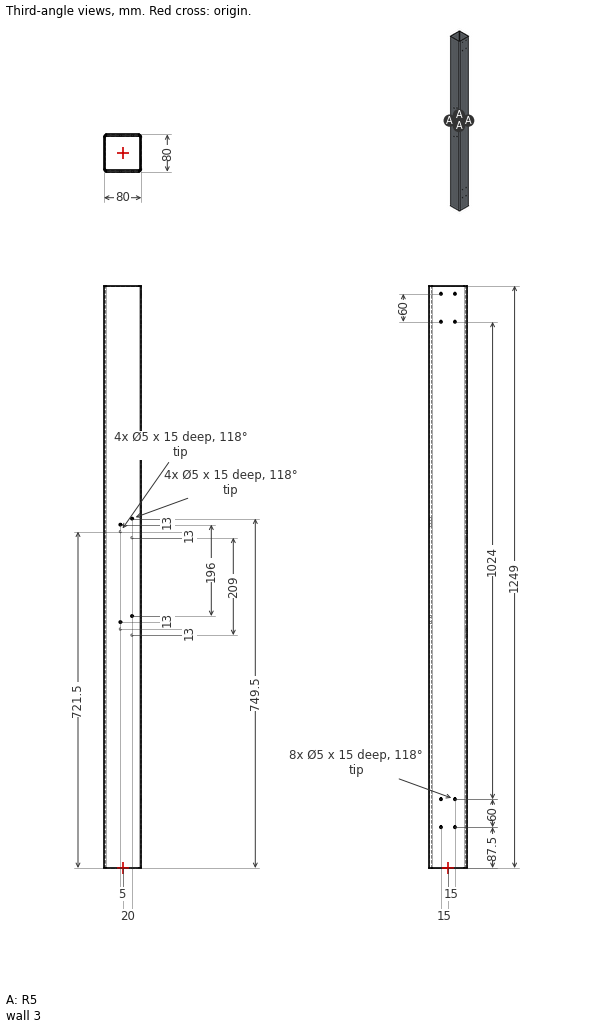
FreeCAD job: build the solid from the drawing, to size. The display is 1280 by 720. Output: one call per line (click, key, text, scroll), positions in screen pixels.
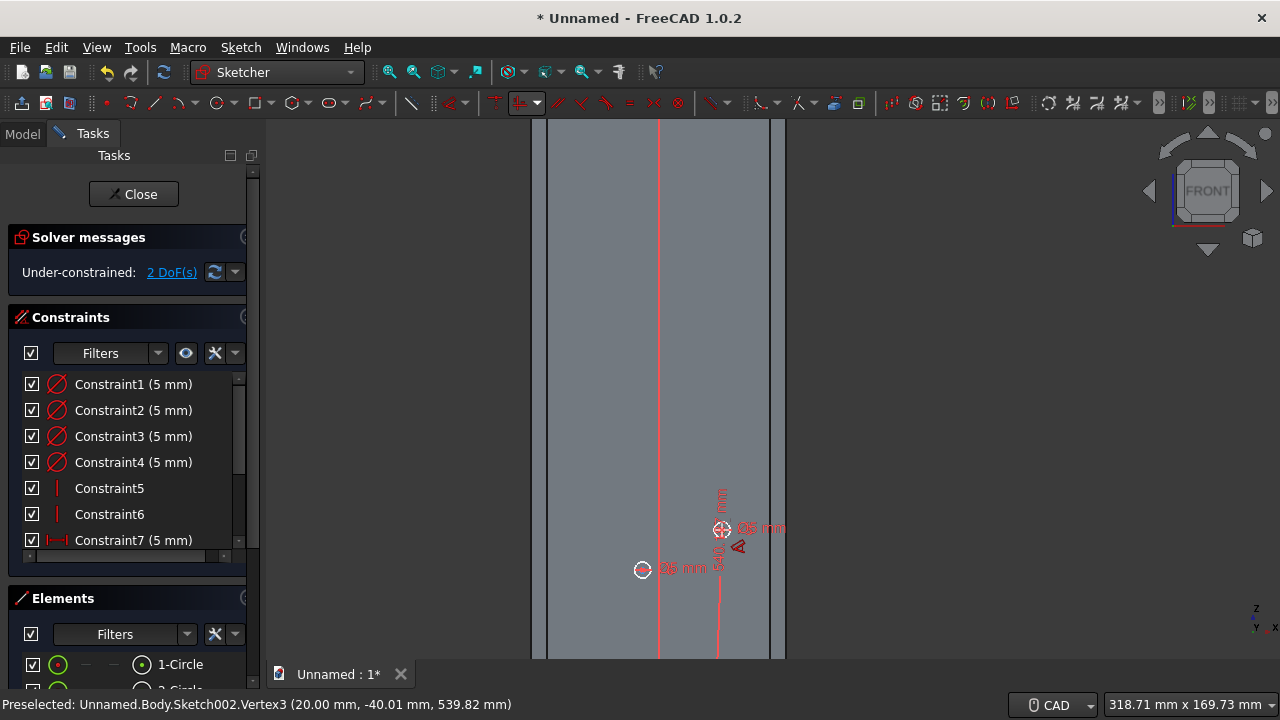
click(643, 570)
click(756, 550)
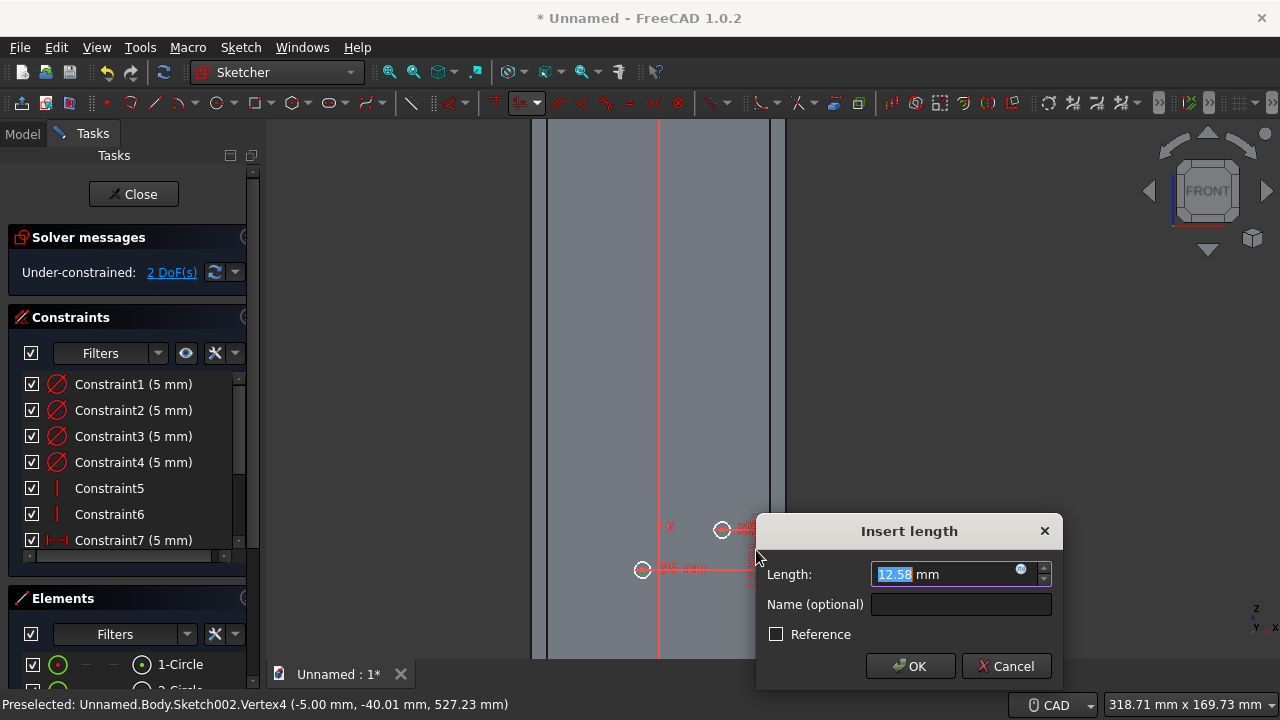
text(13)
key(Return)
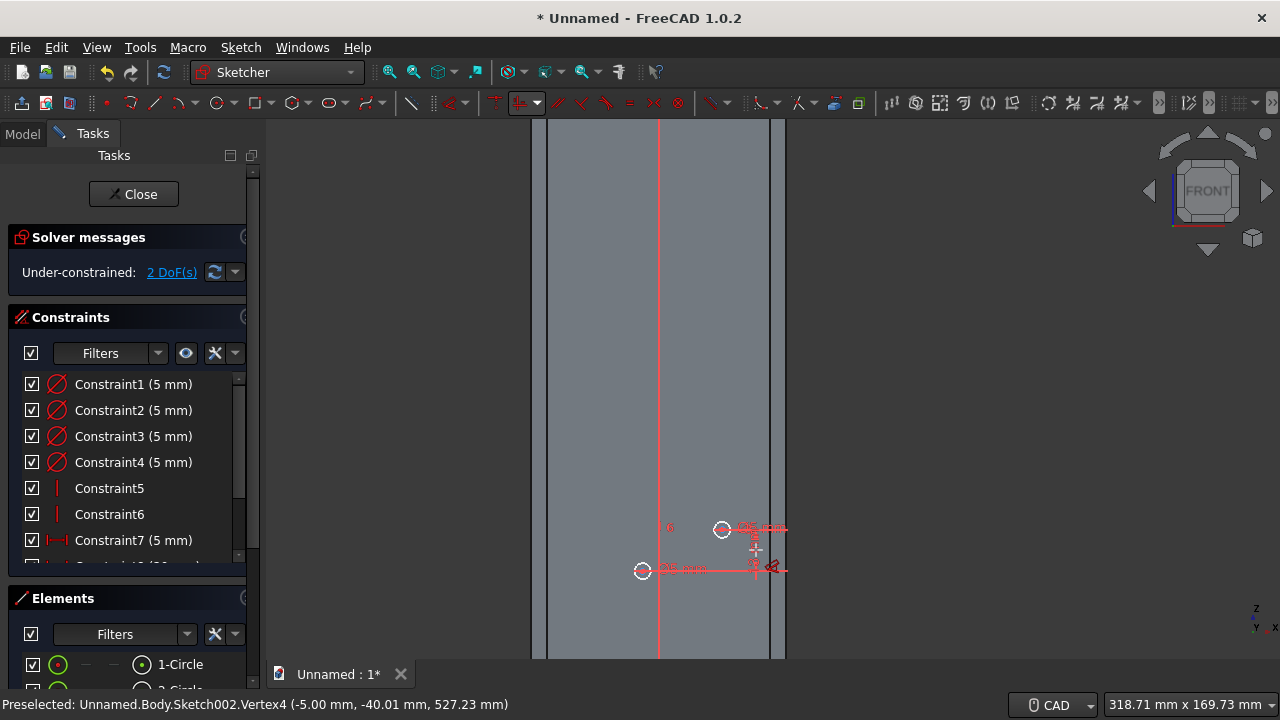
scroll(723, 530, down, 4)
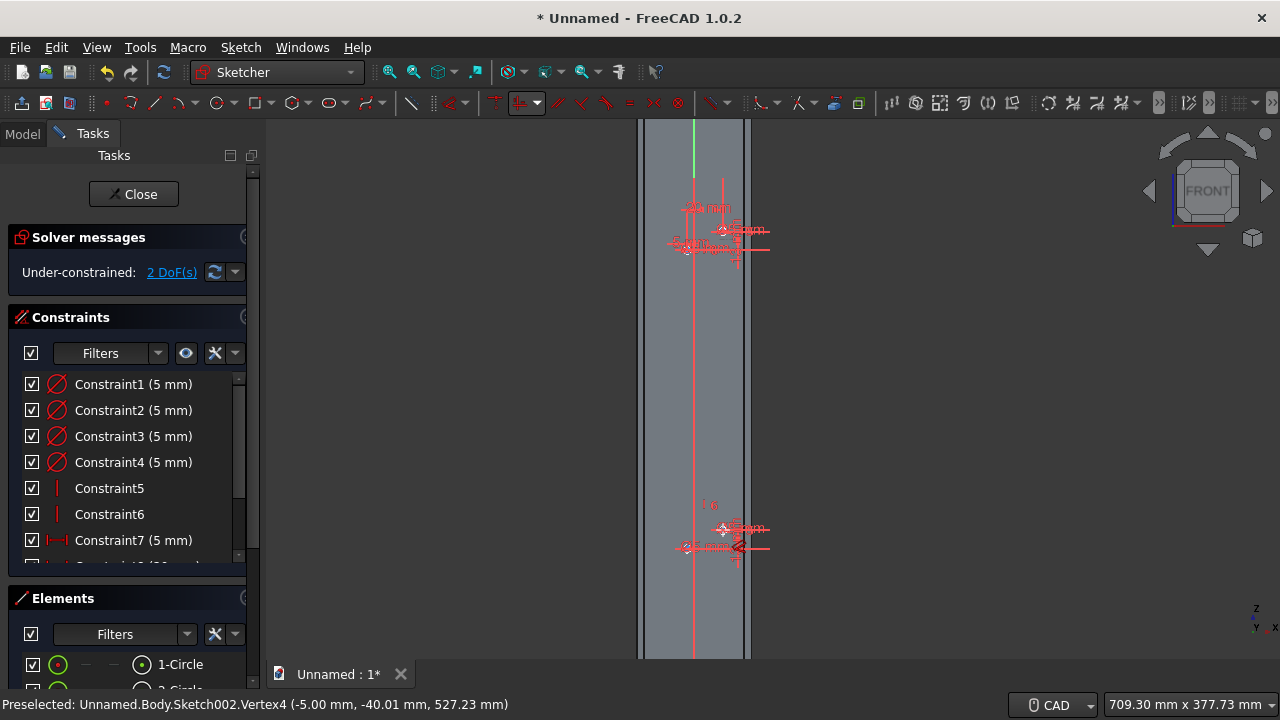
click(687, 250)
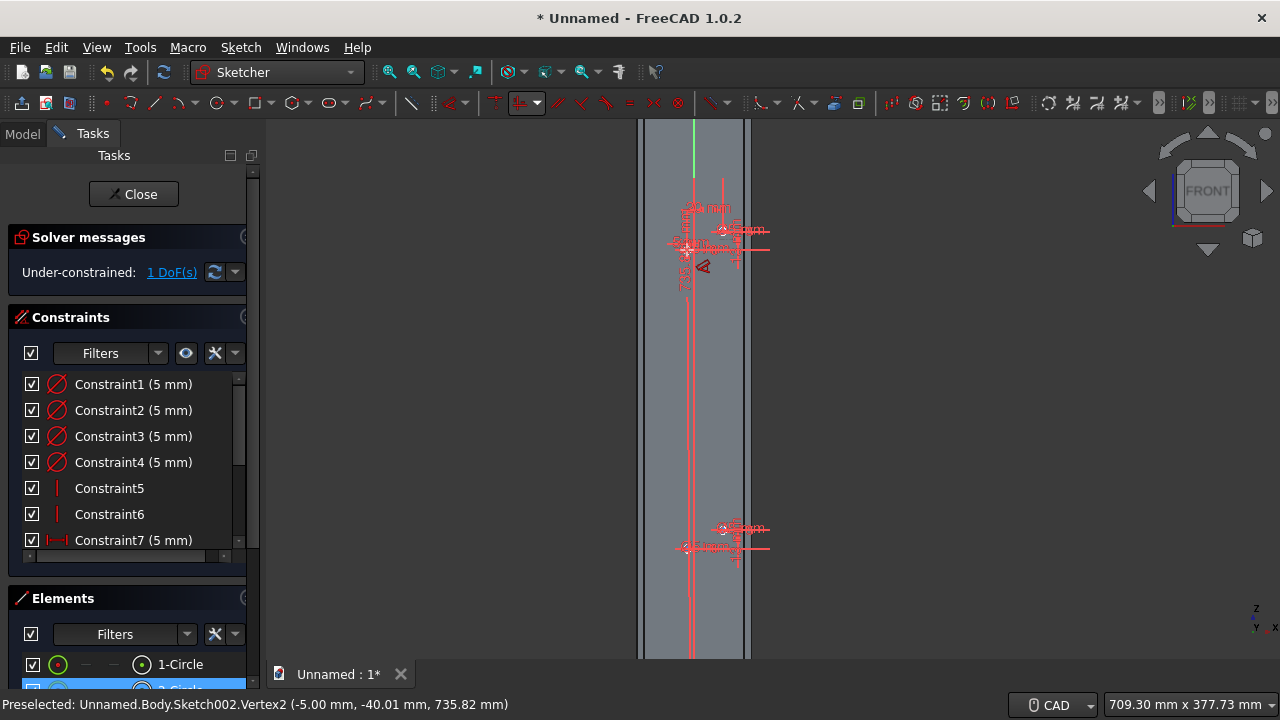
click(723, 530)
click(757, 390)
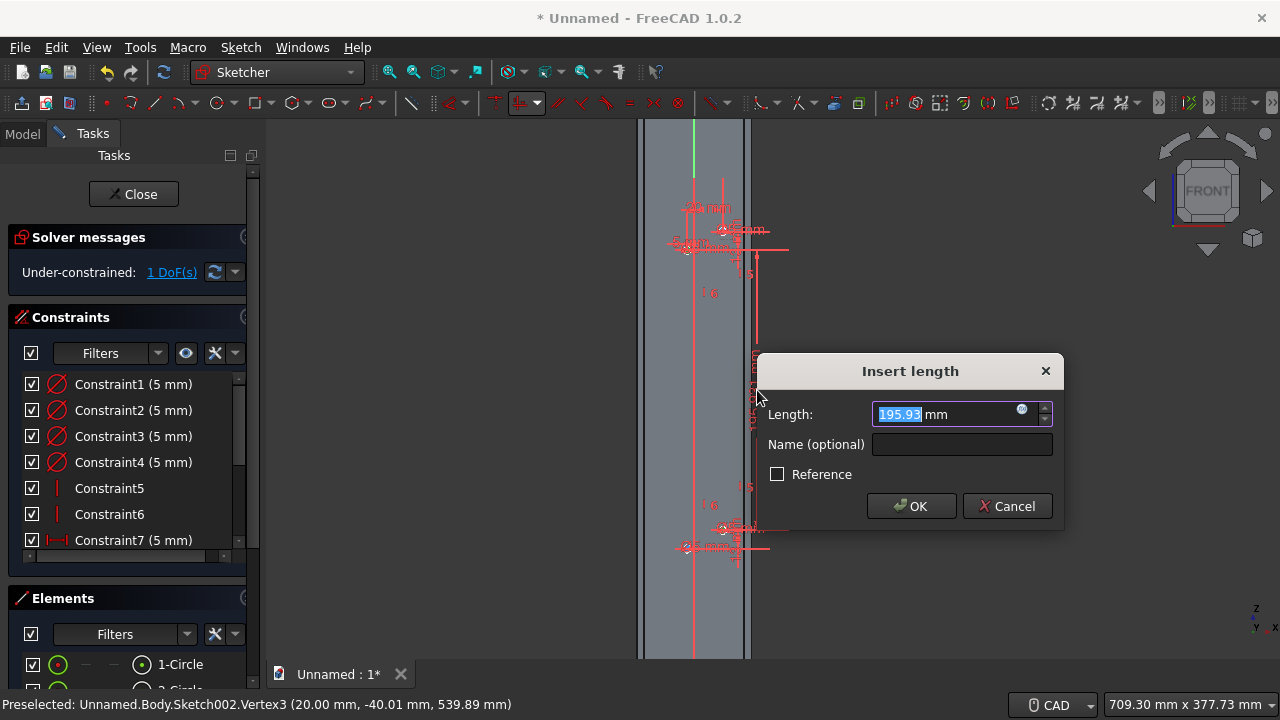
text(196)
key(Return)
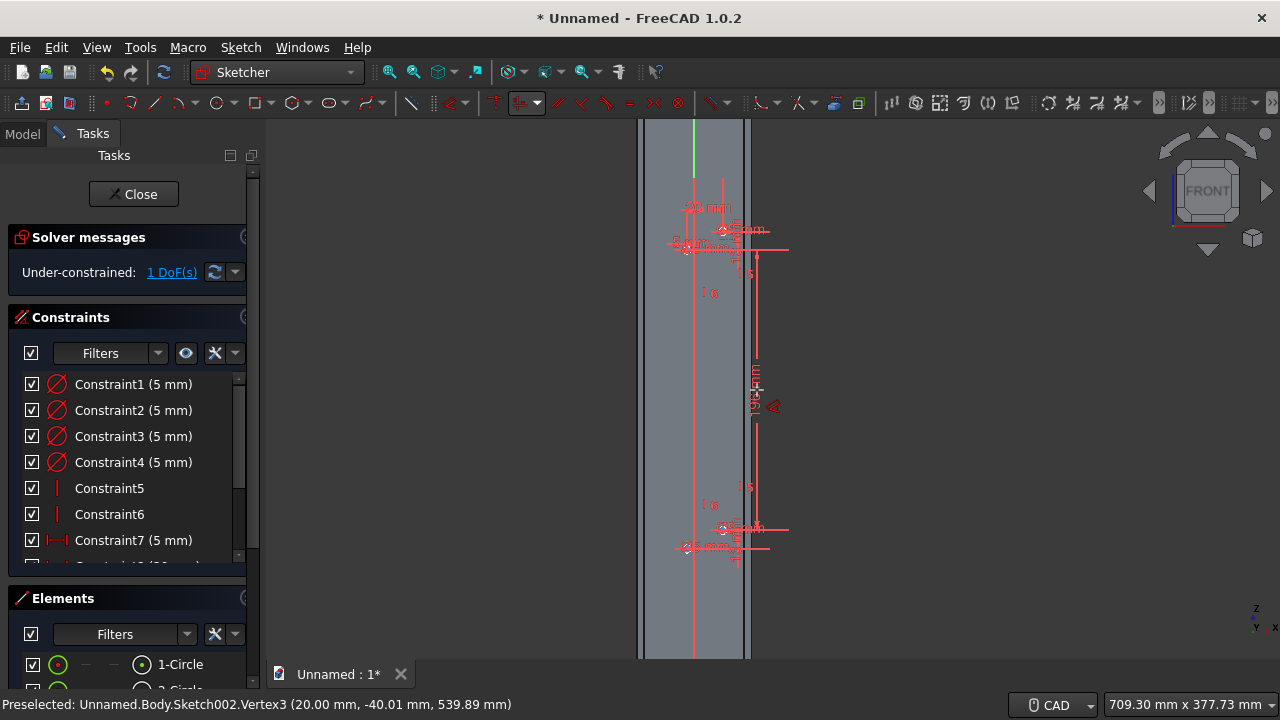
click(723, 232)
click(757, 431)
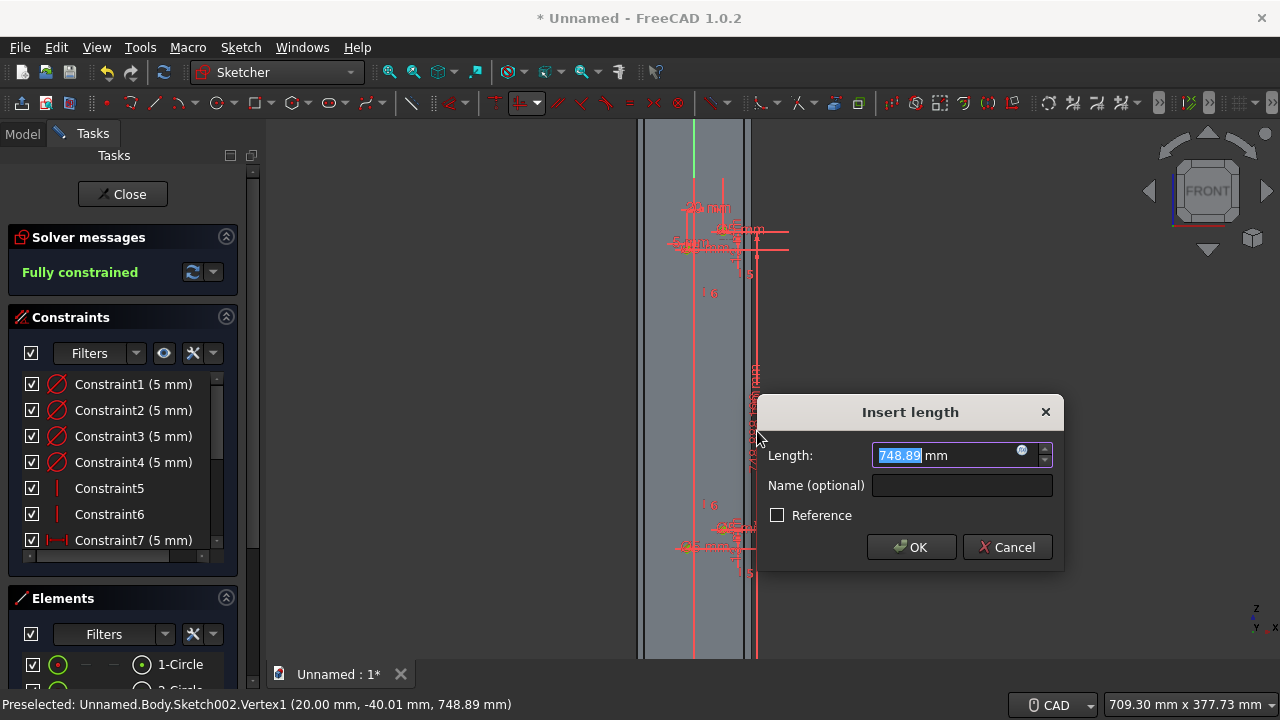
text(749.5)
key(Return)
key(Escape)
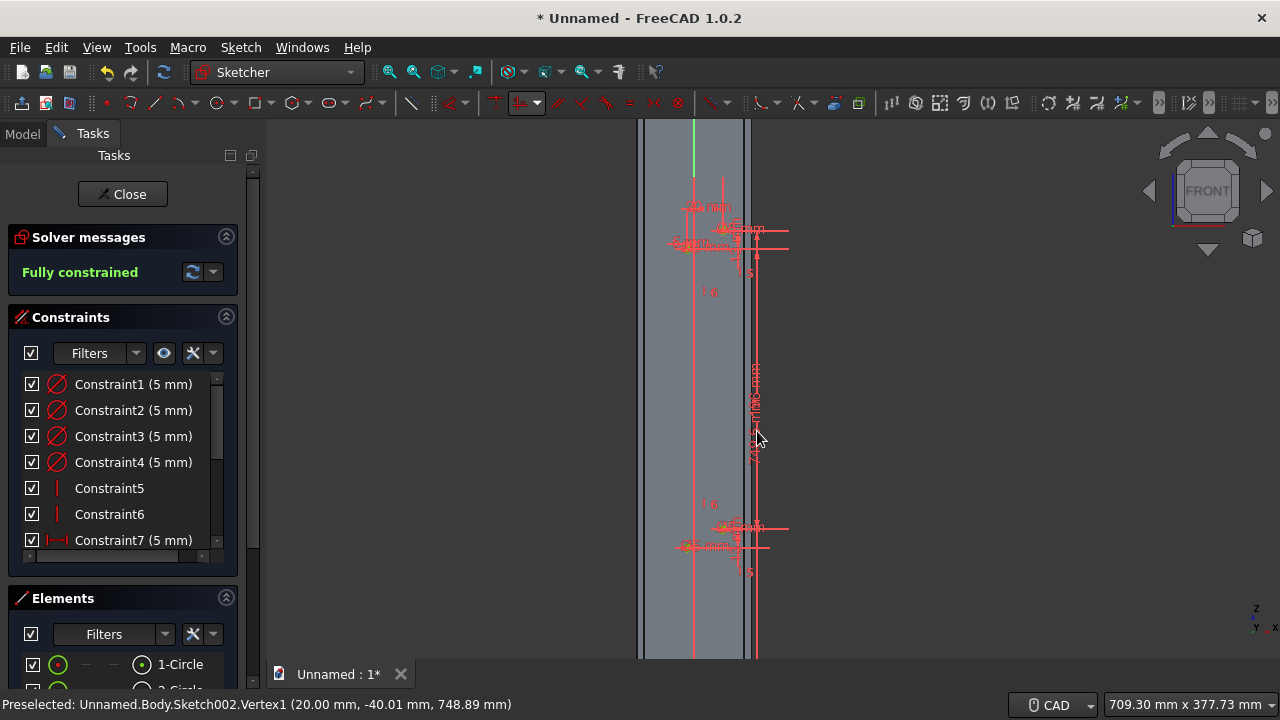
click(123, 194)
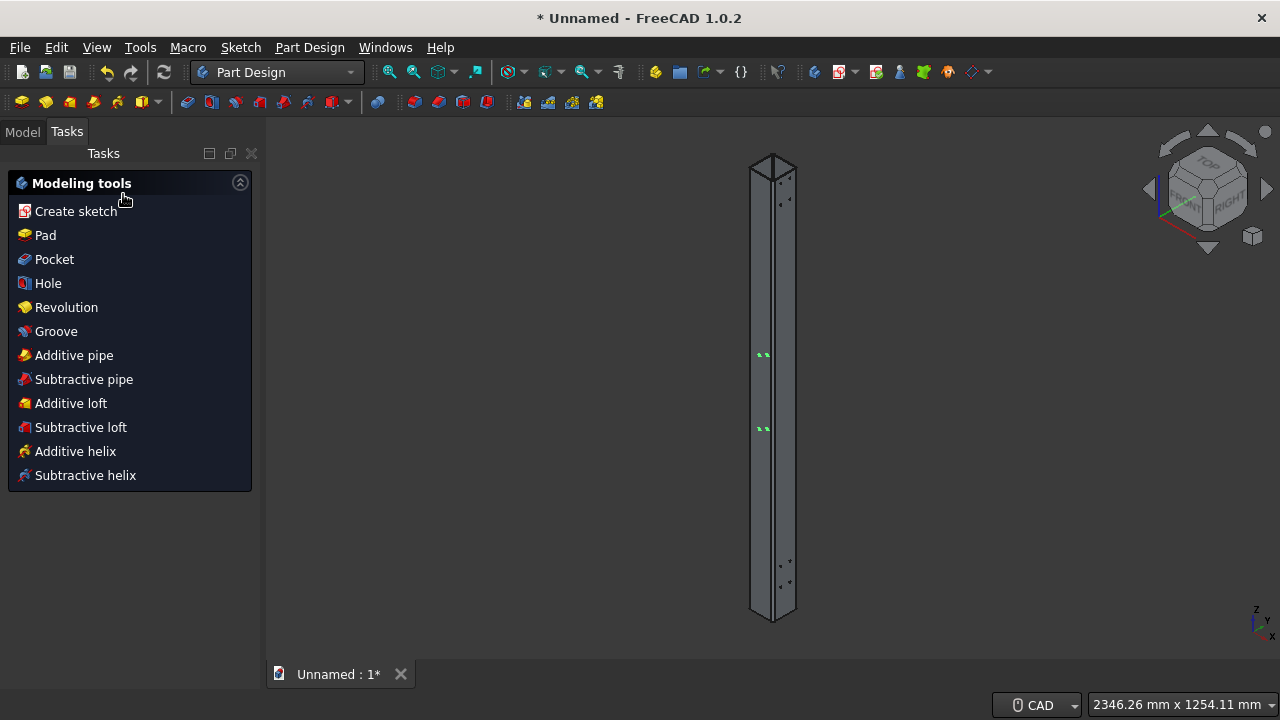
click(212, 102)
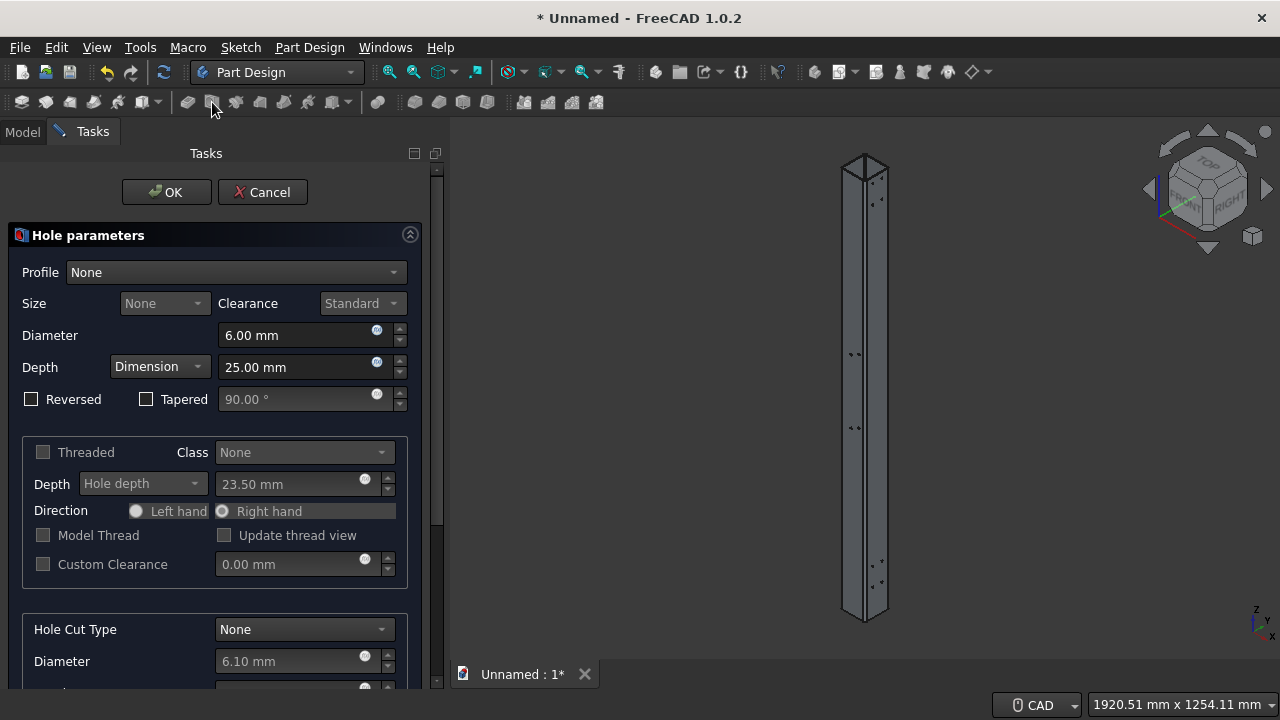
triple_click(305, 335)